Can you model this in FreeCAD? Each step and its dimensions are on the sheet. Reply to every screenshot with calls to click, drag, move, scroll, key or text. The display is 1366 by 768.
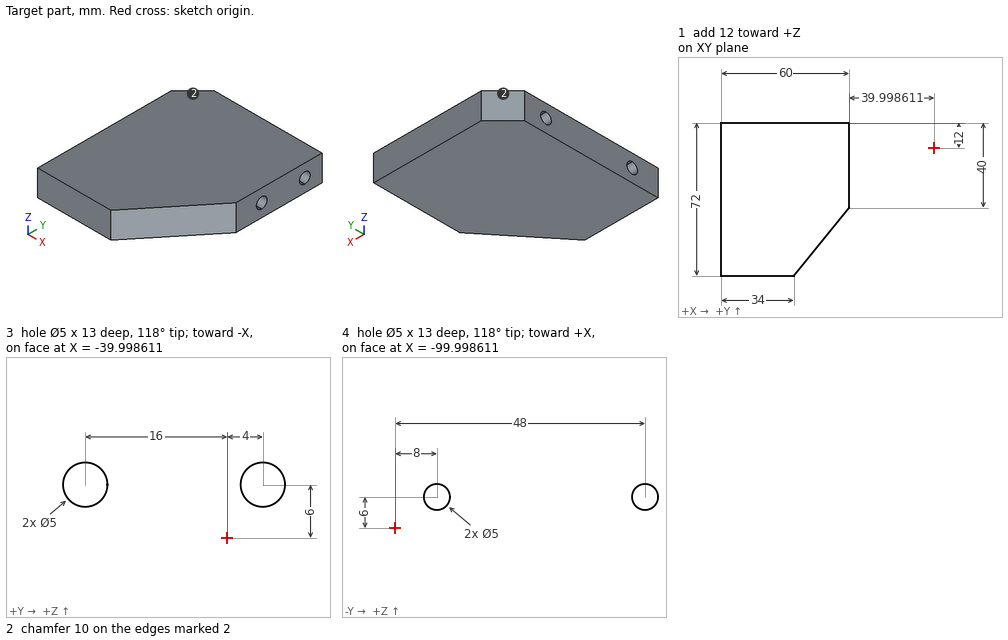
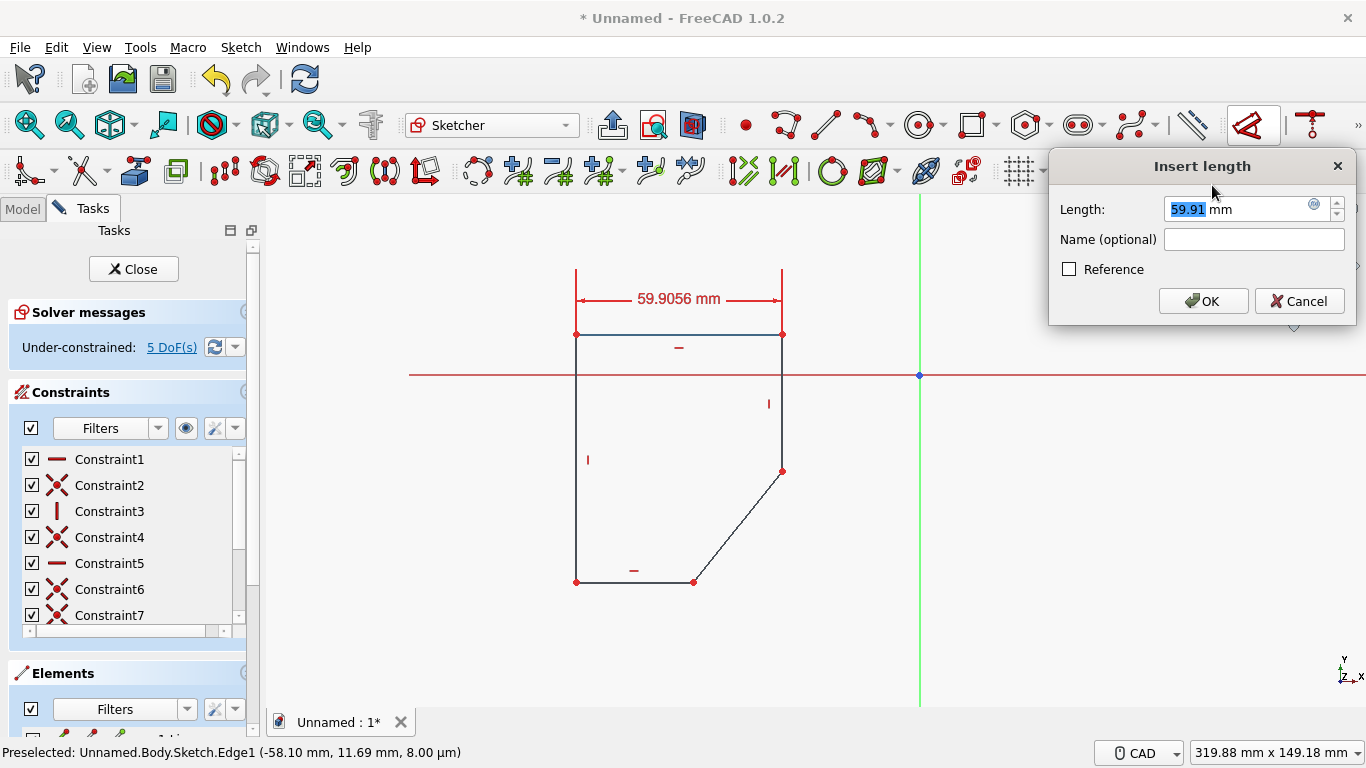
text(60)
key(Return)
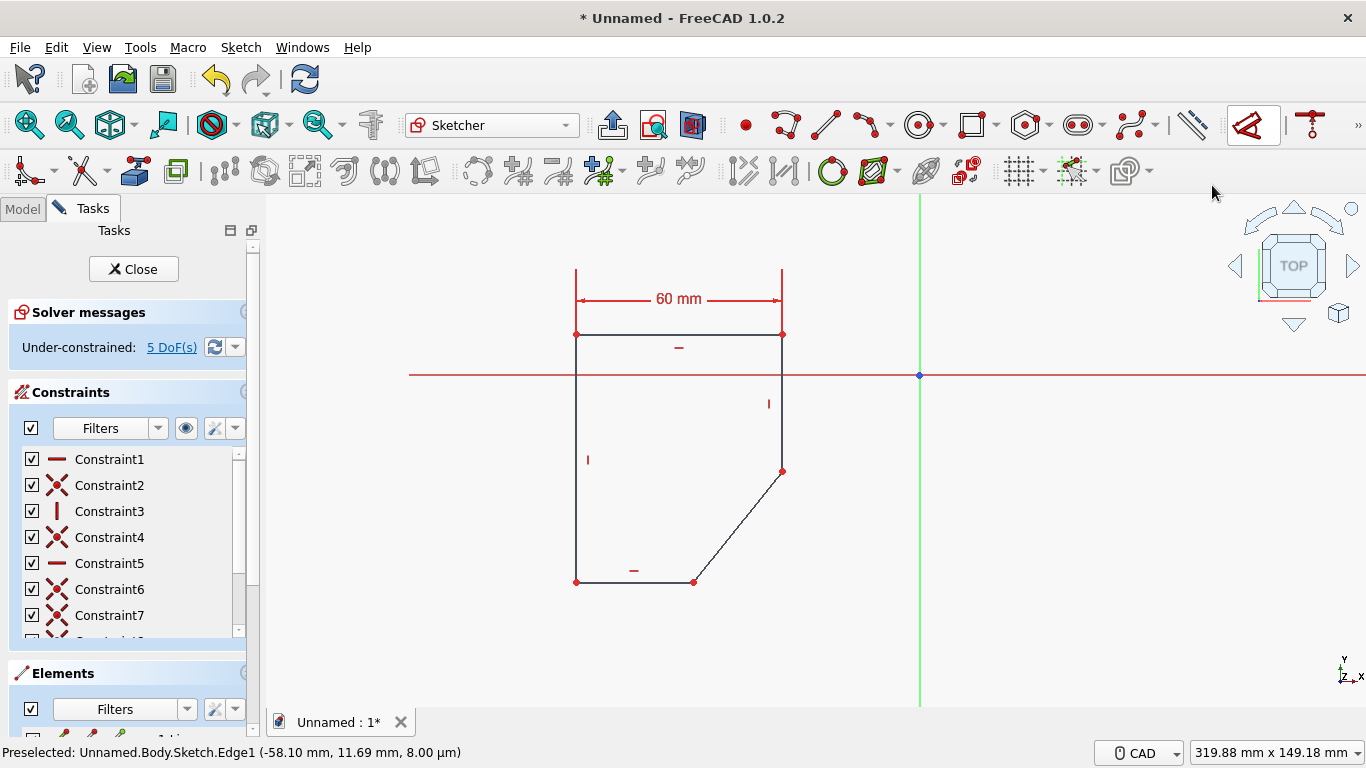
click(576, 409)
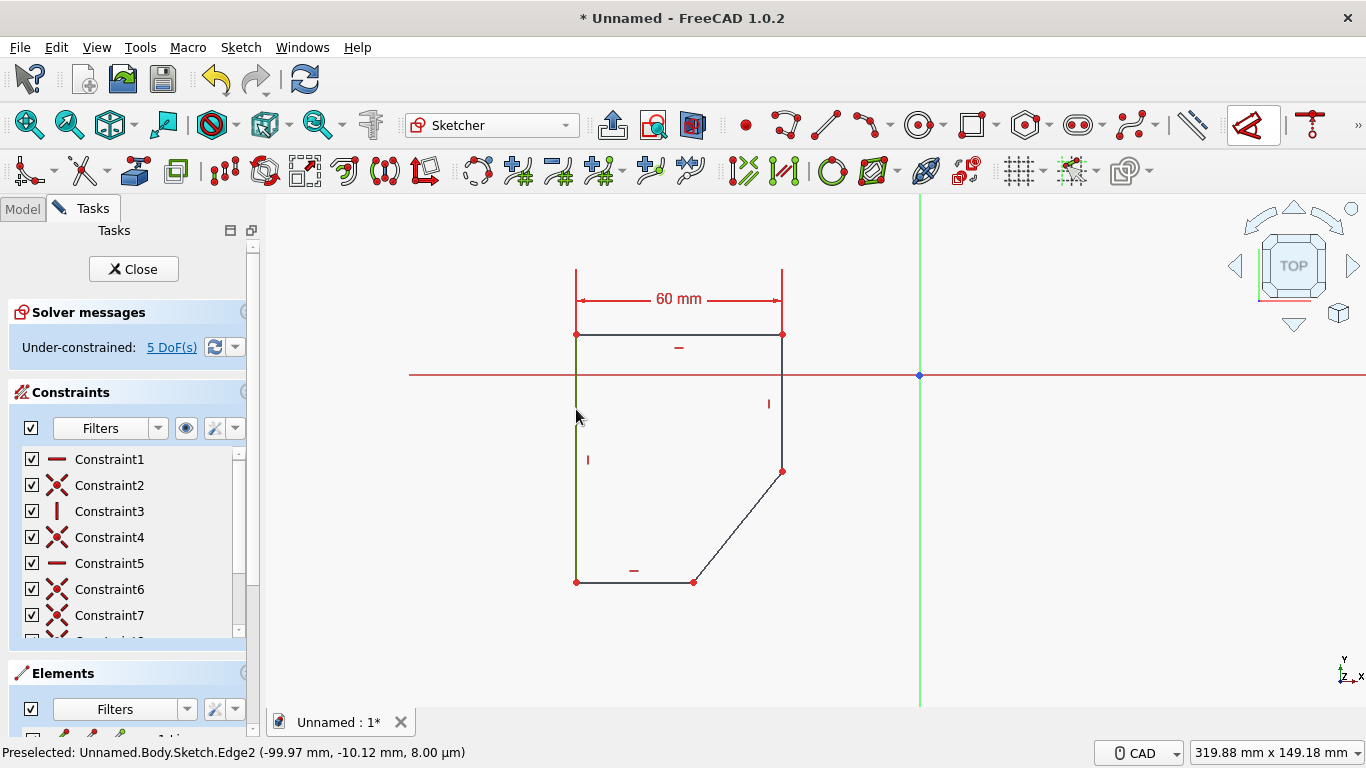
key(i)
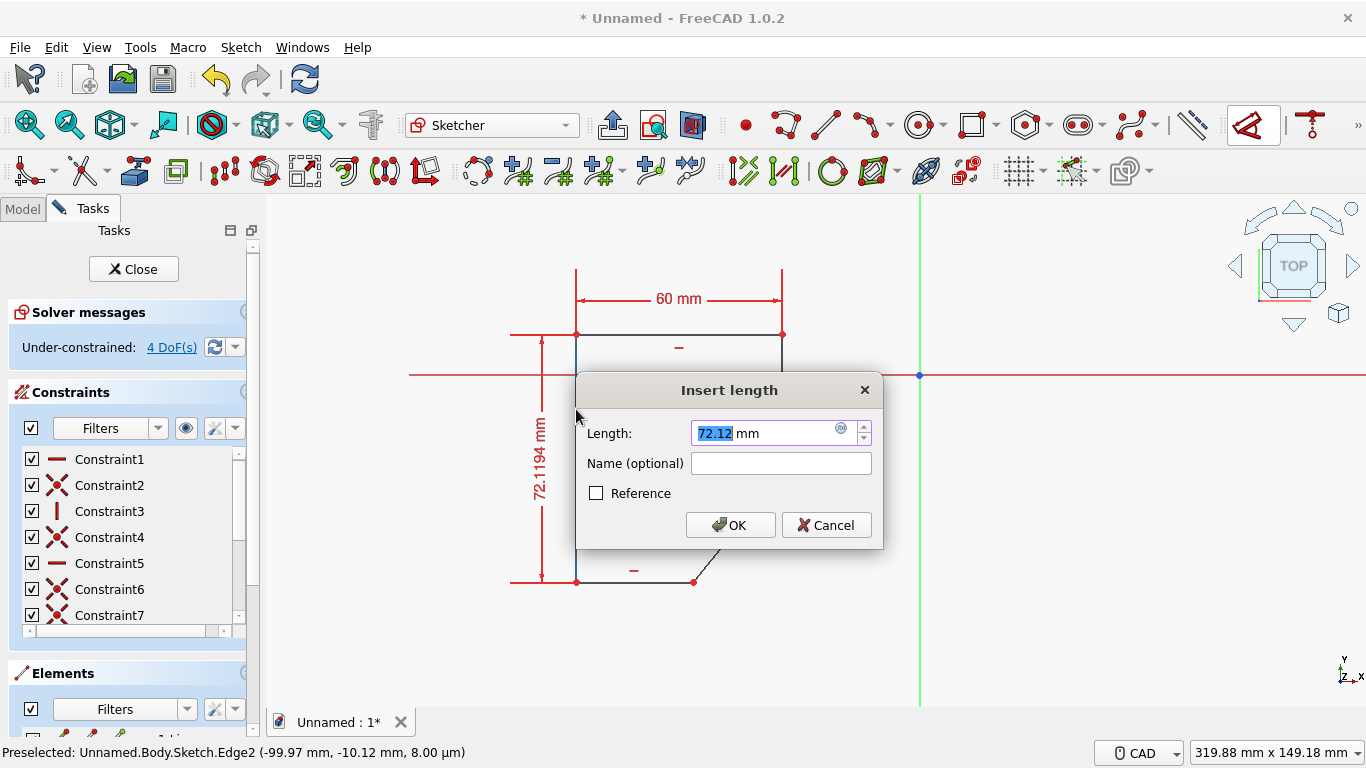
text(72)
key(Return)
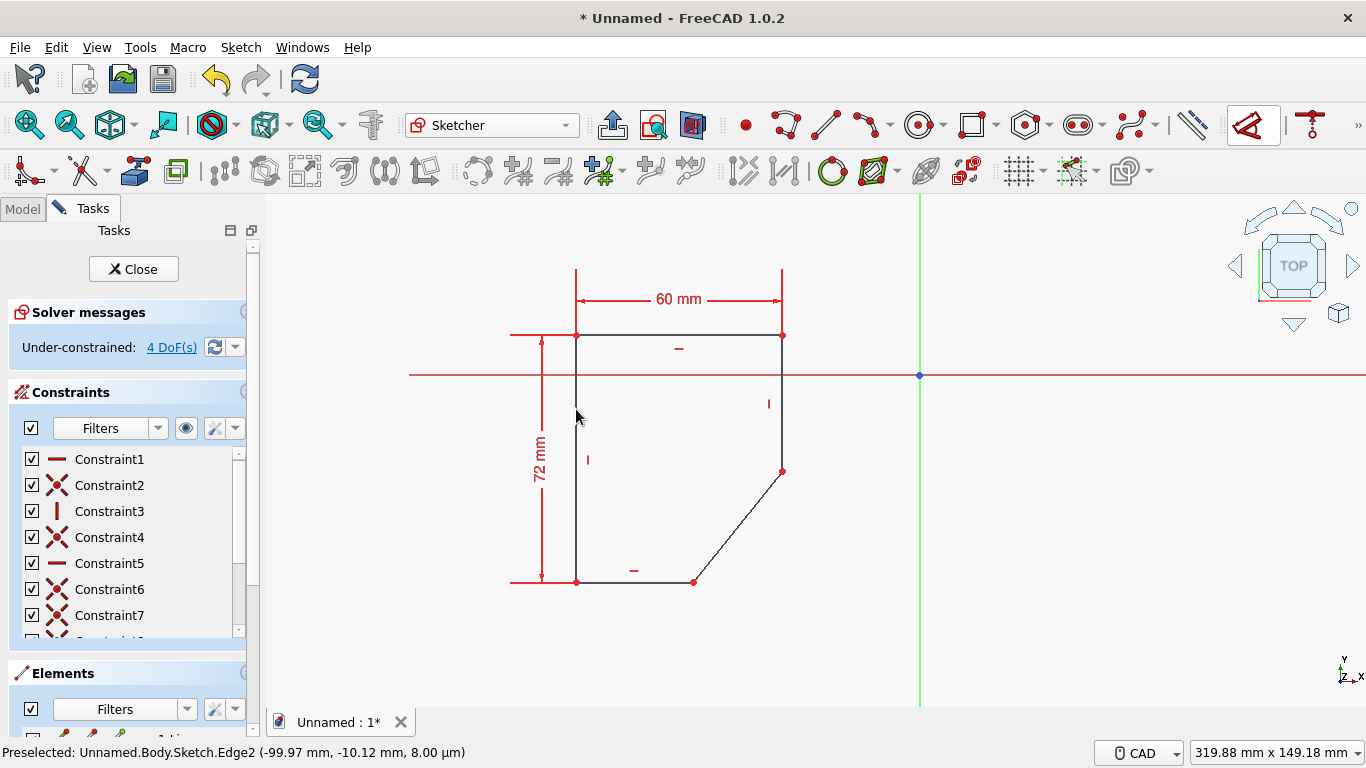
click(611, 583)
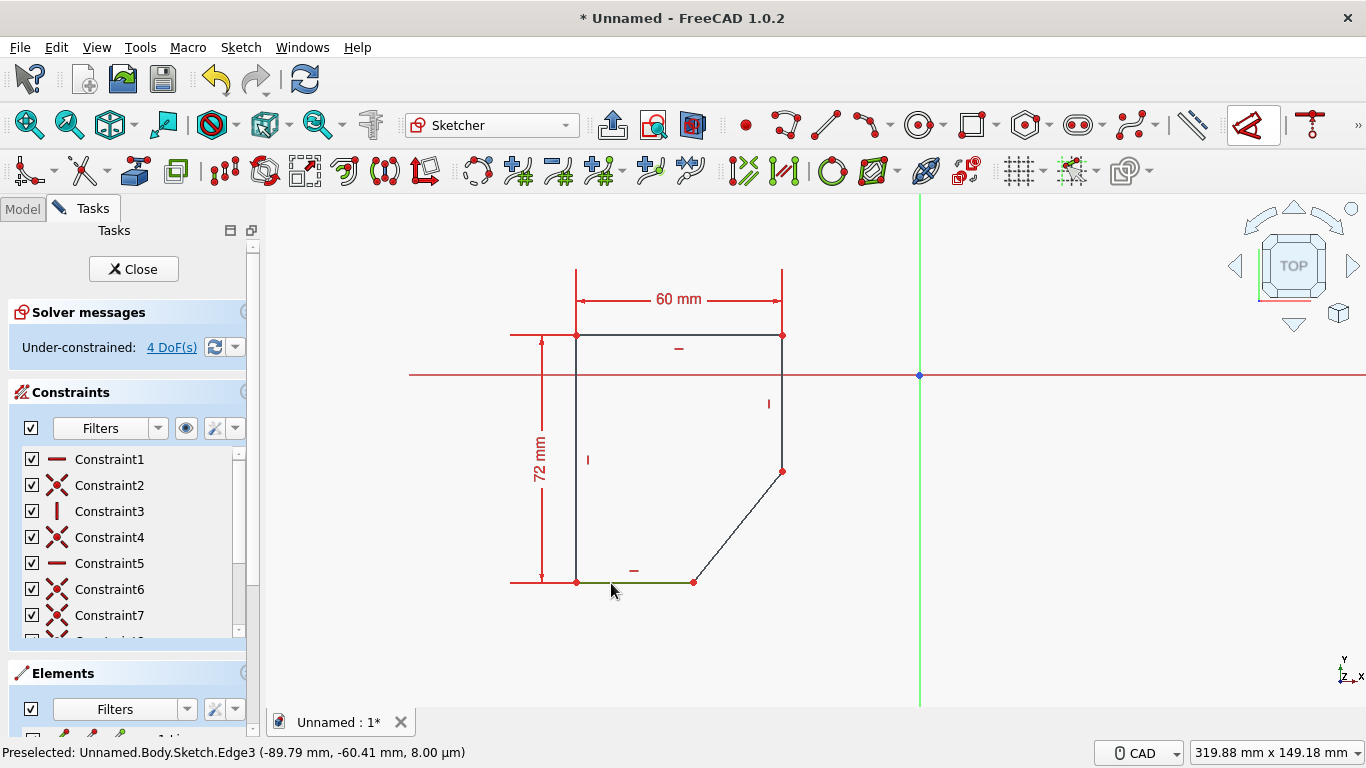
key(l)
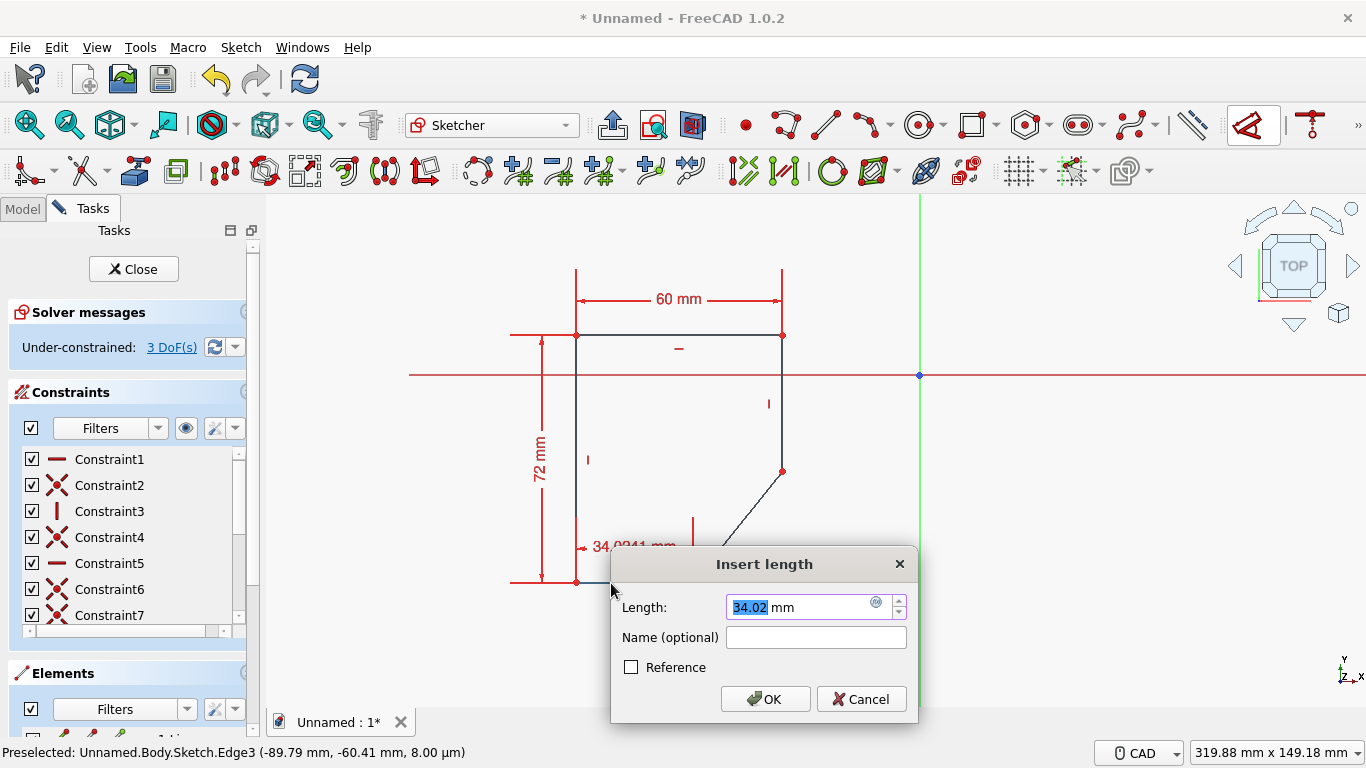
text(34)
key(Return)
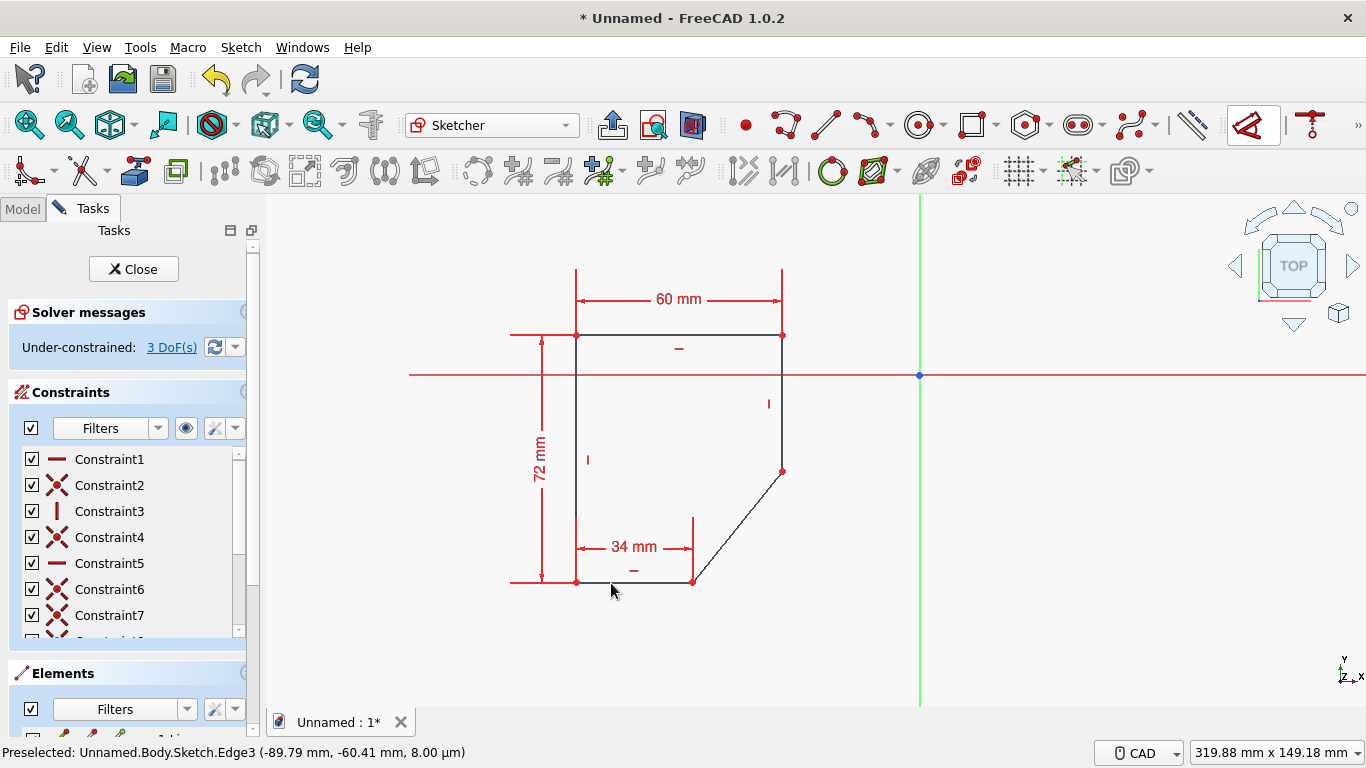
click(782, 431)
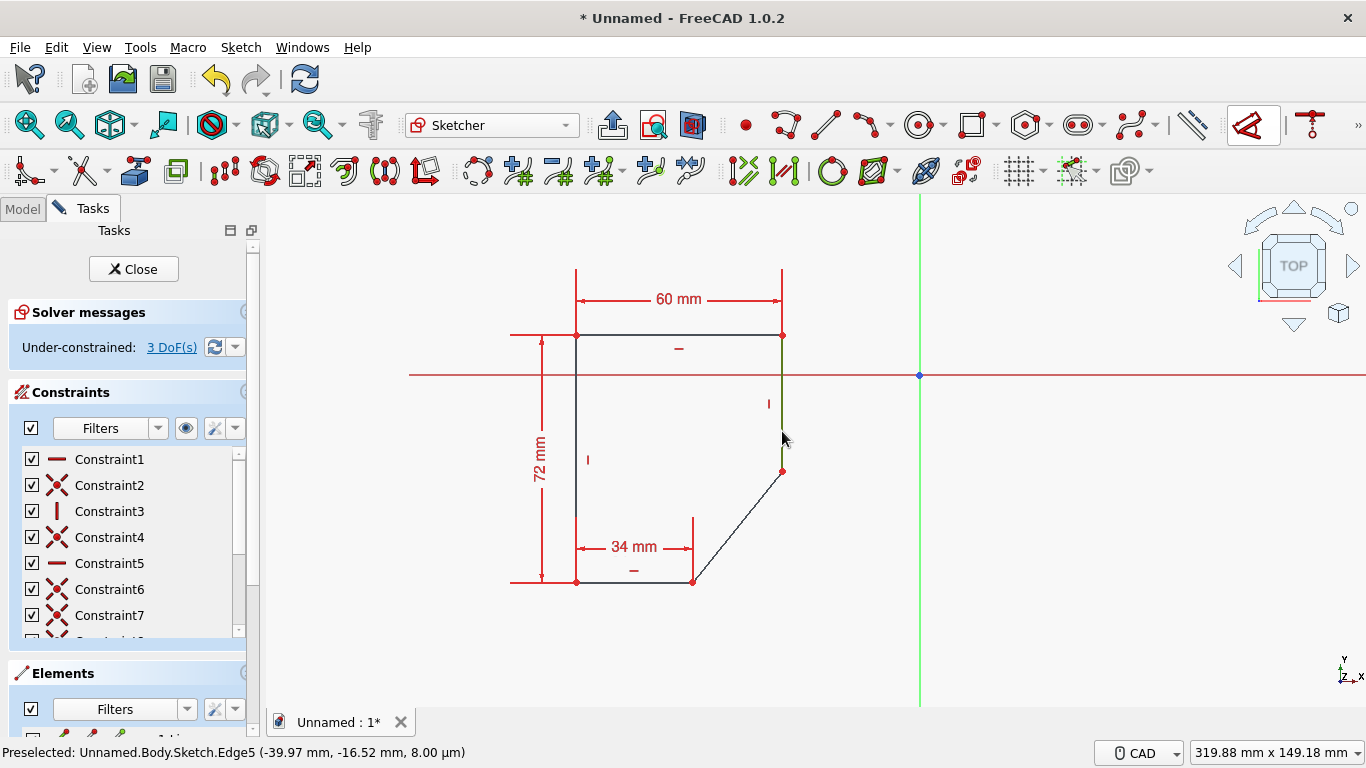
click(1274, 126)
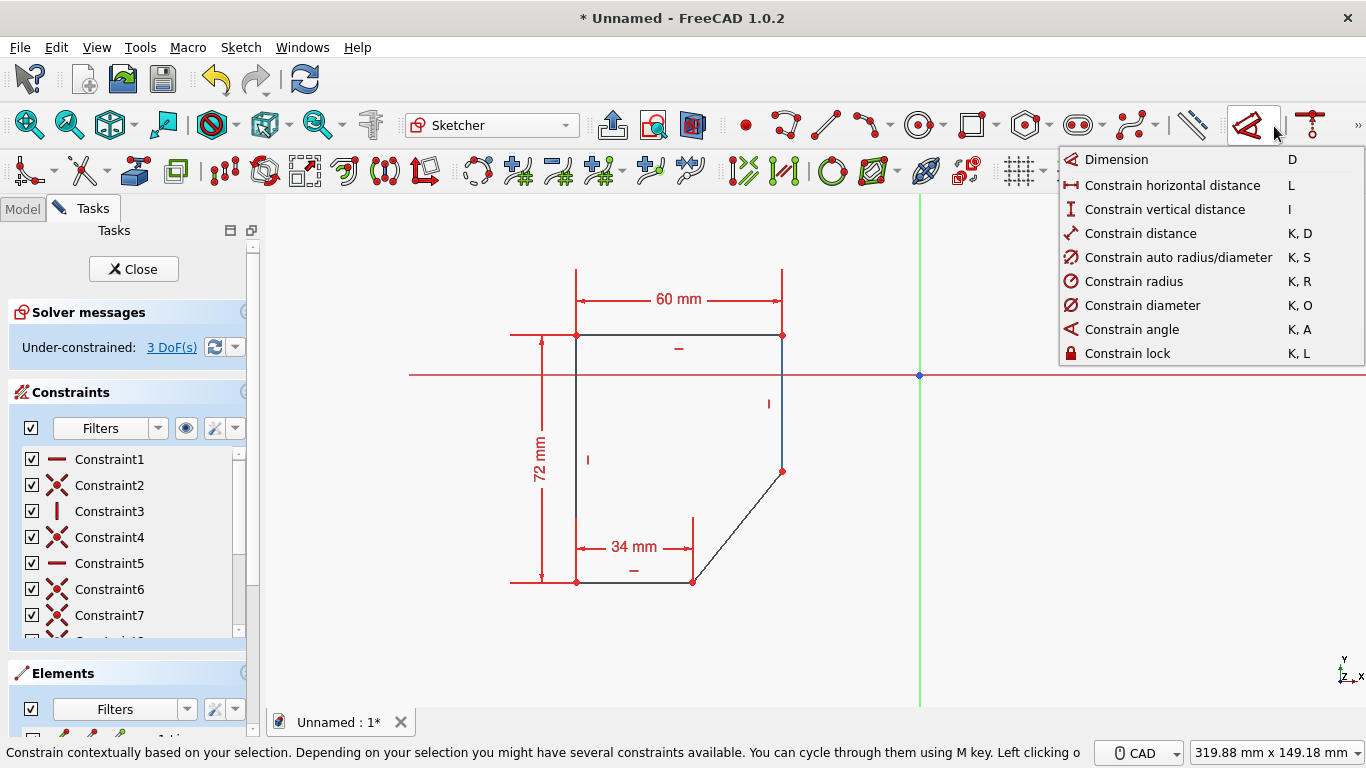
click(1212, 209)